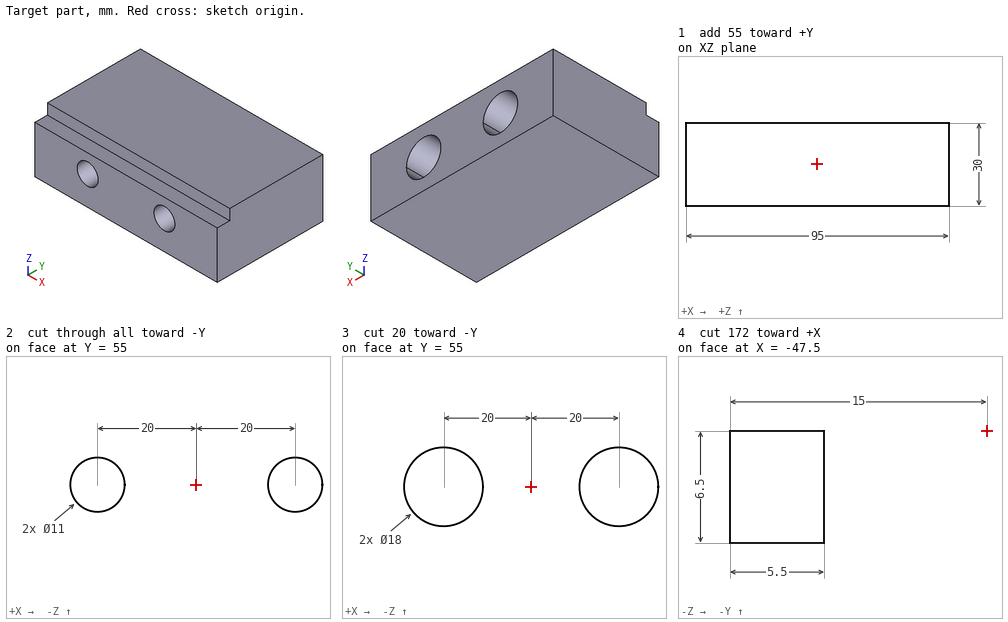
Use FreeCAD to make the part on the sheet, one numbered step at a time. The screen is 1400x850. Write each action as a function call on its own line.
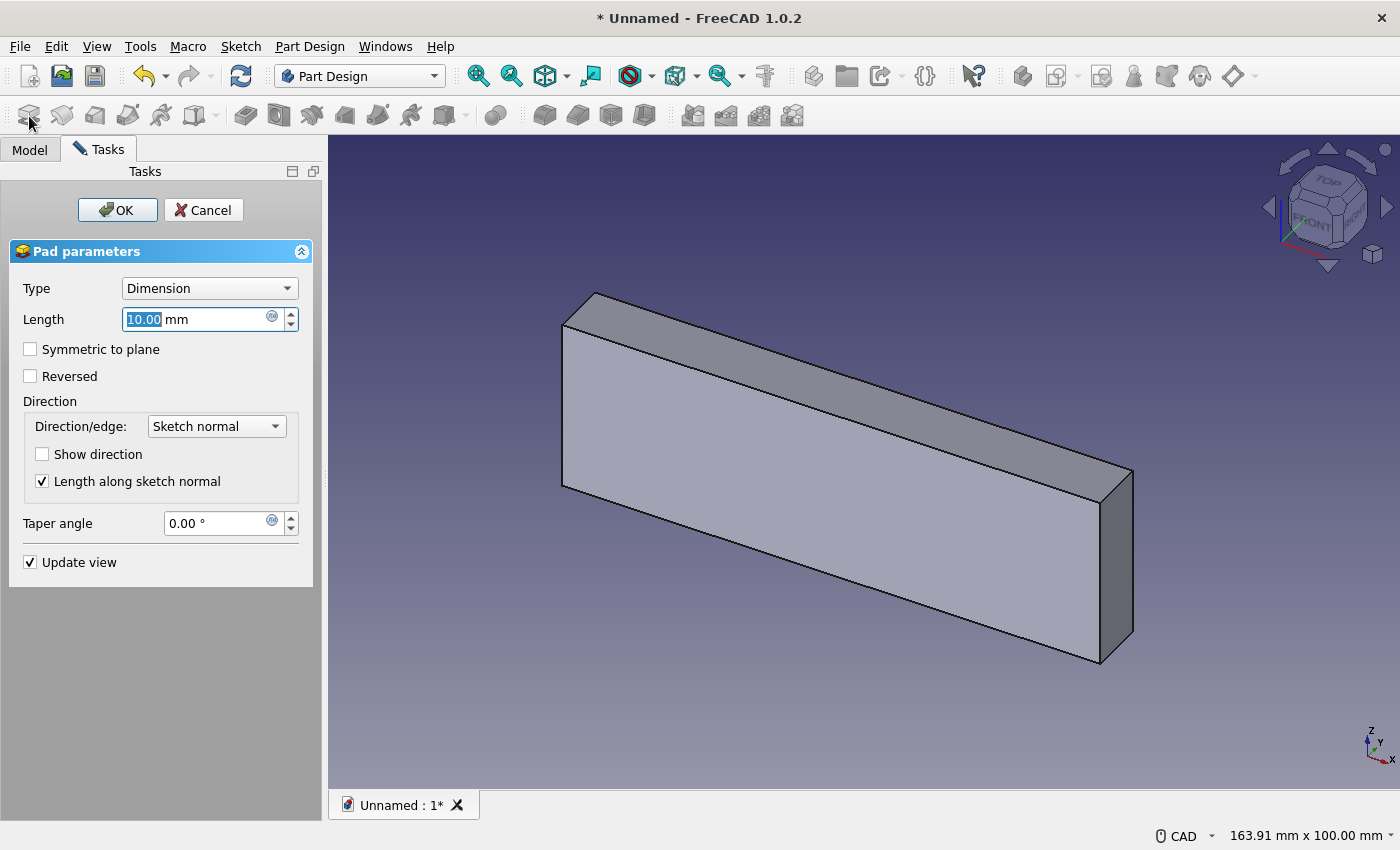
text(55)
key(Tab)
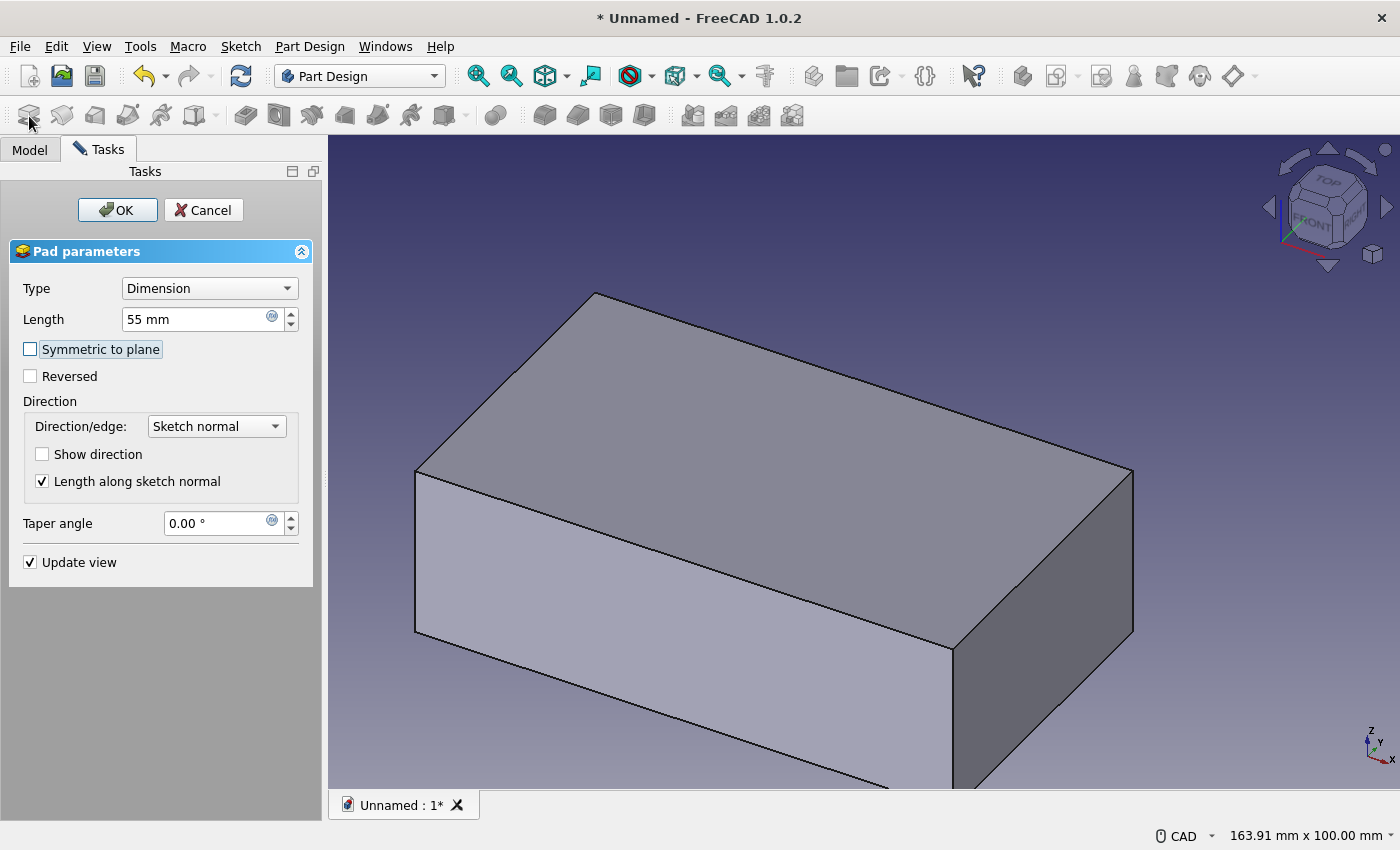
click(31, 376)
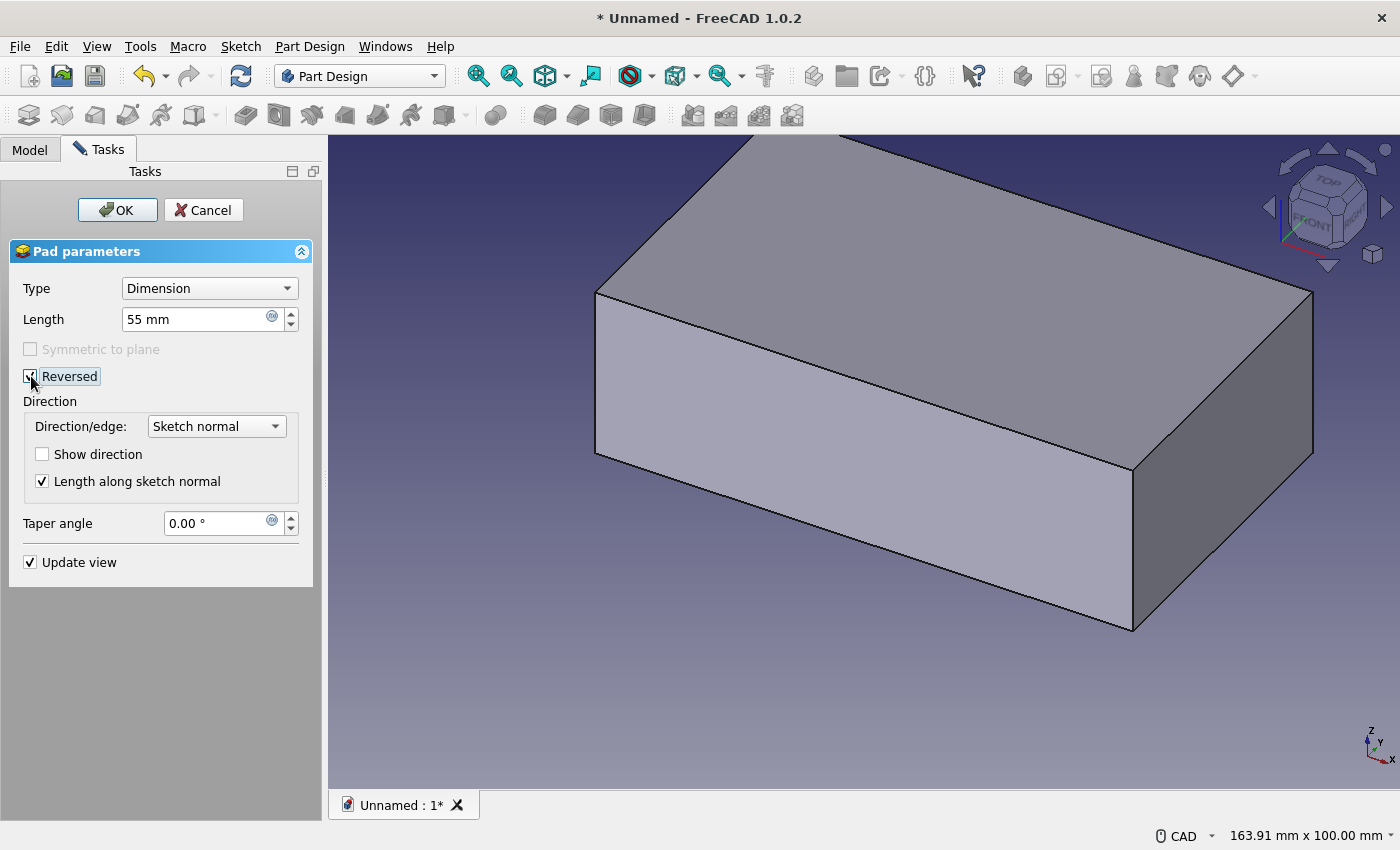
click(118, 210)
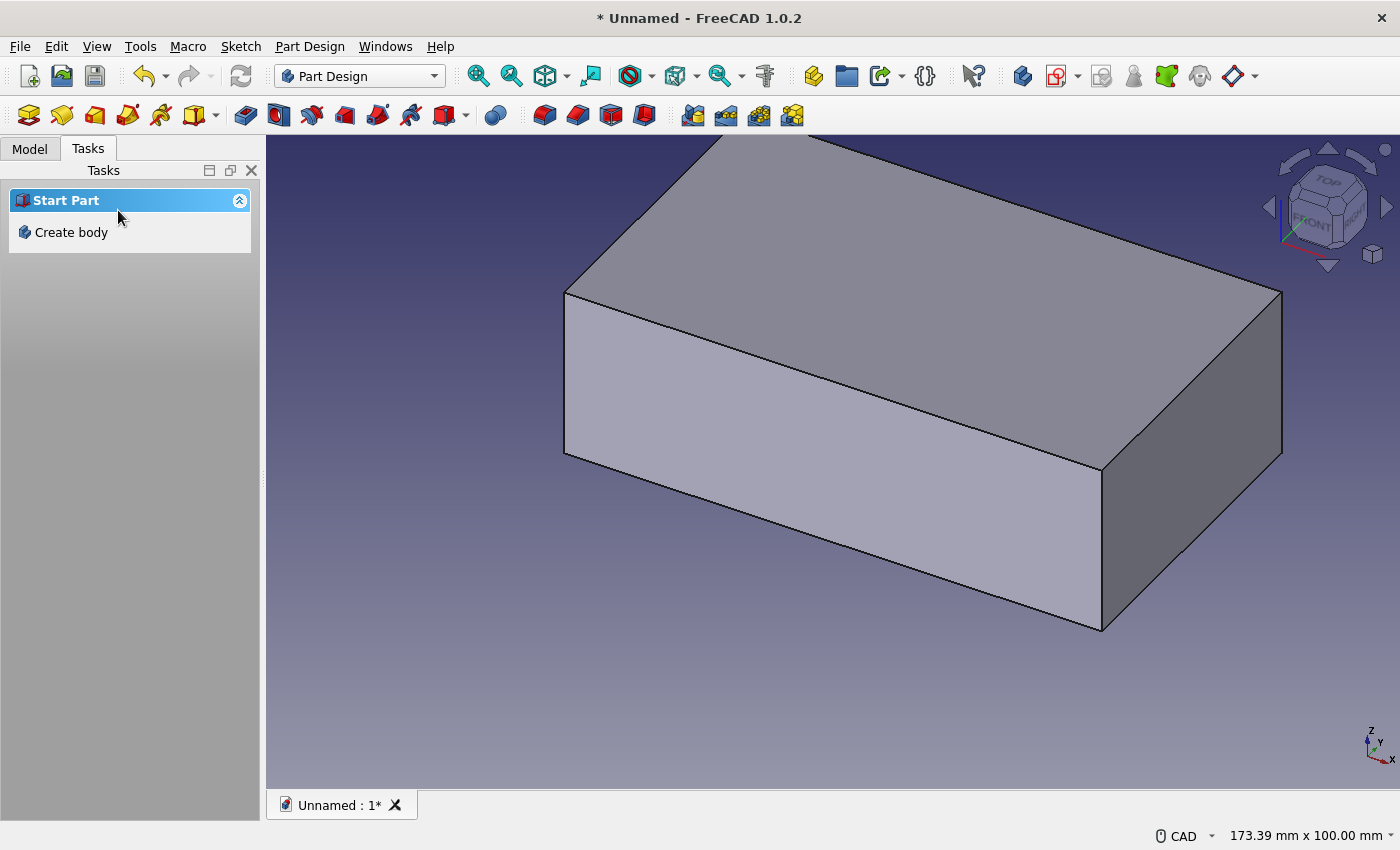
click(479, 76)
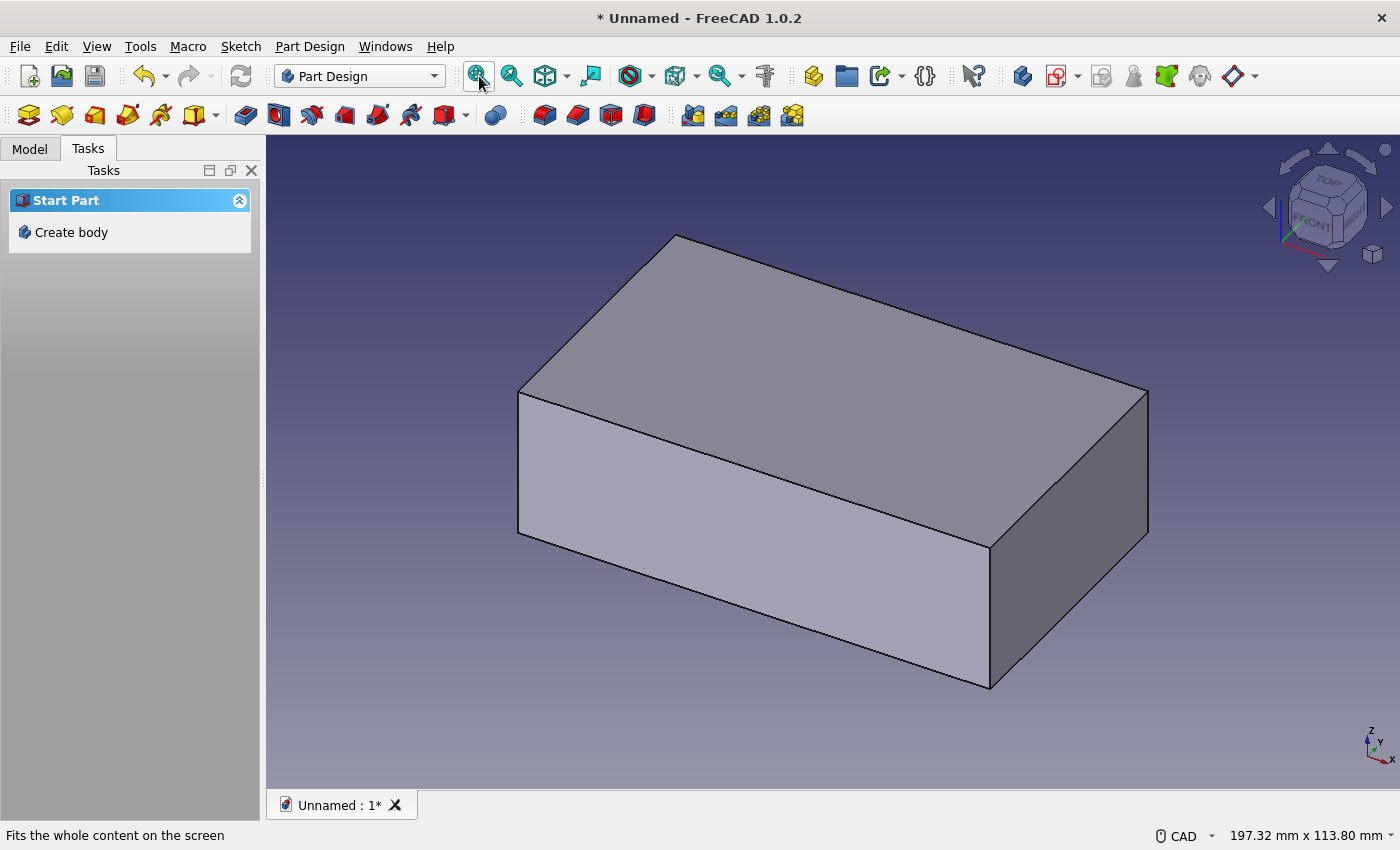
key(4)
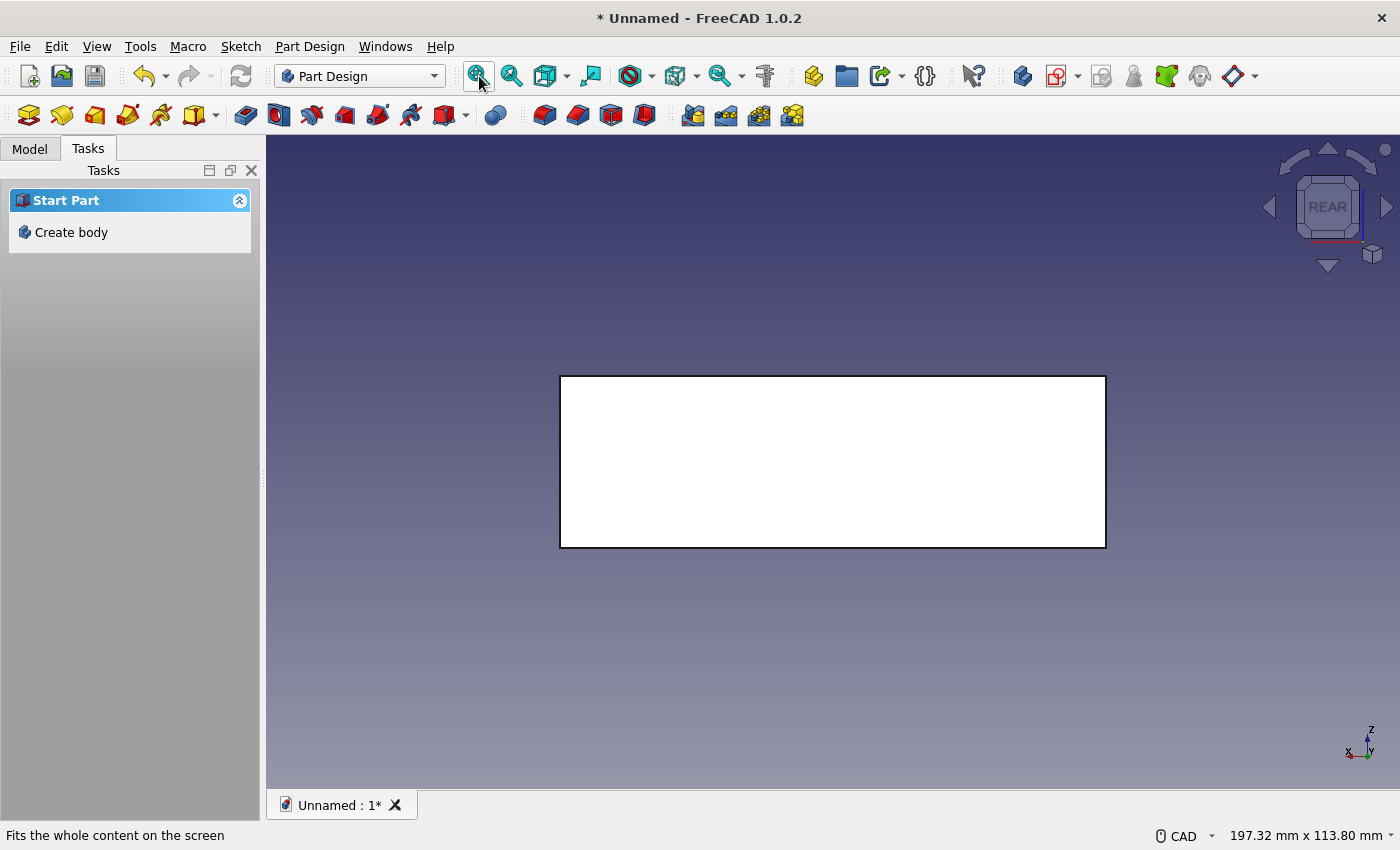
click(677, 461)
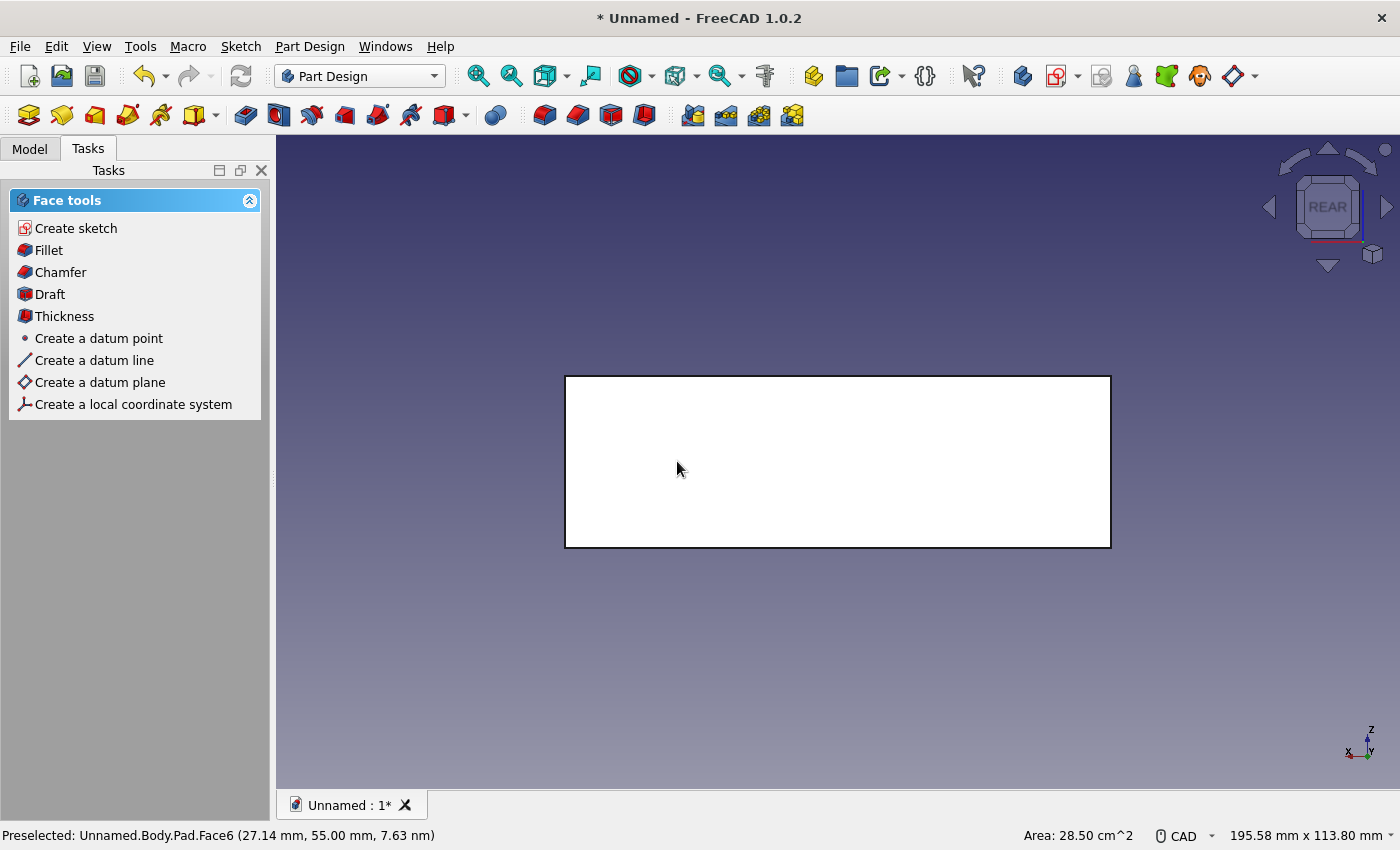
click(1056, 76)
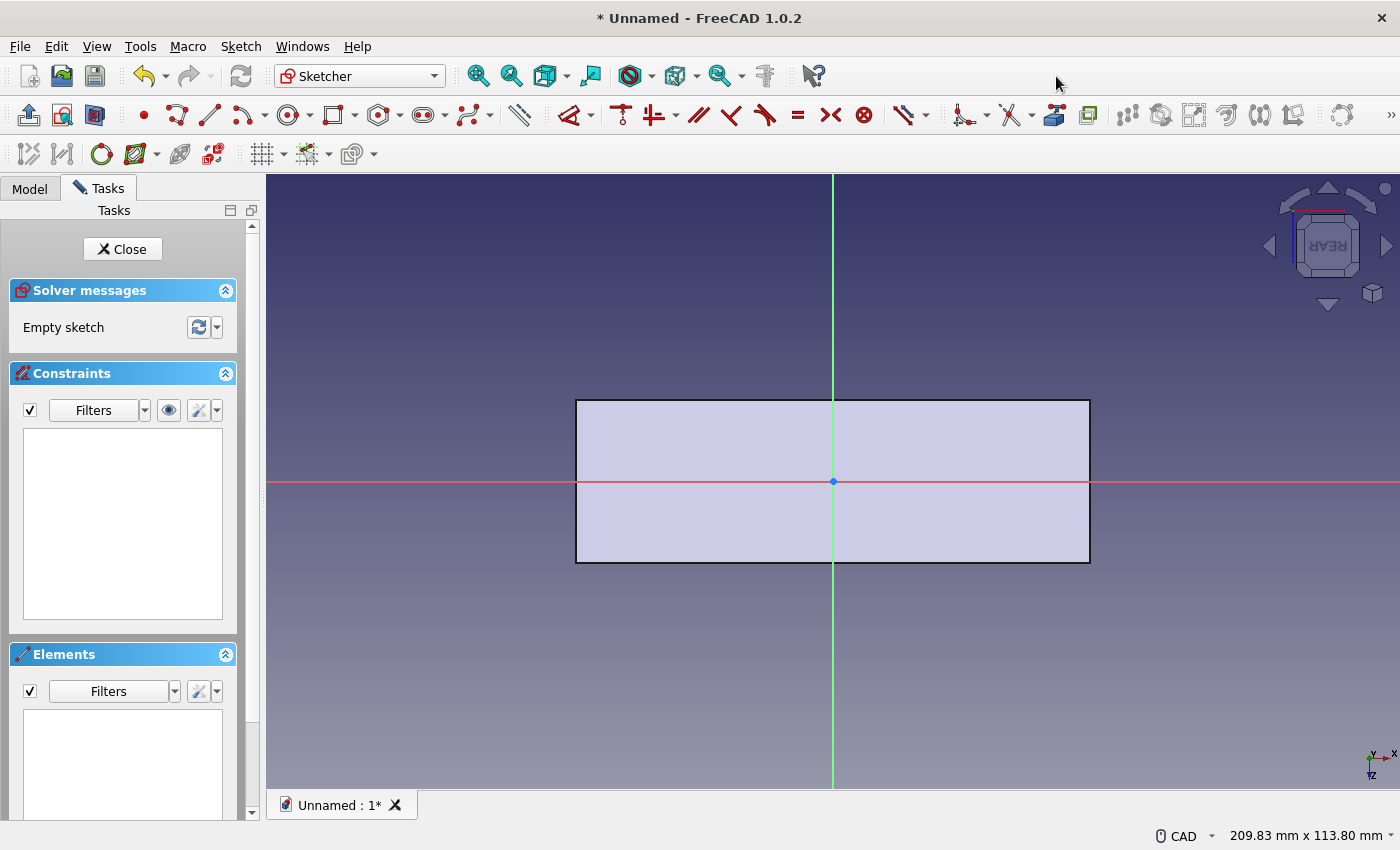
scroll(889, 481, up, 4)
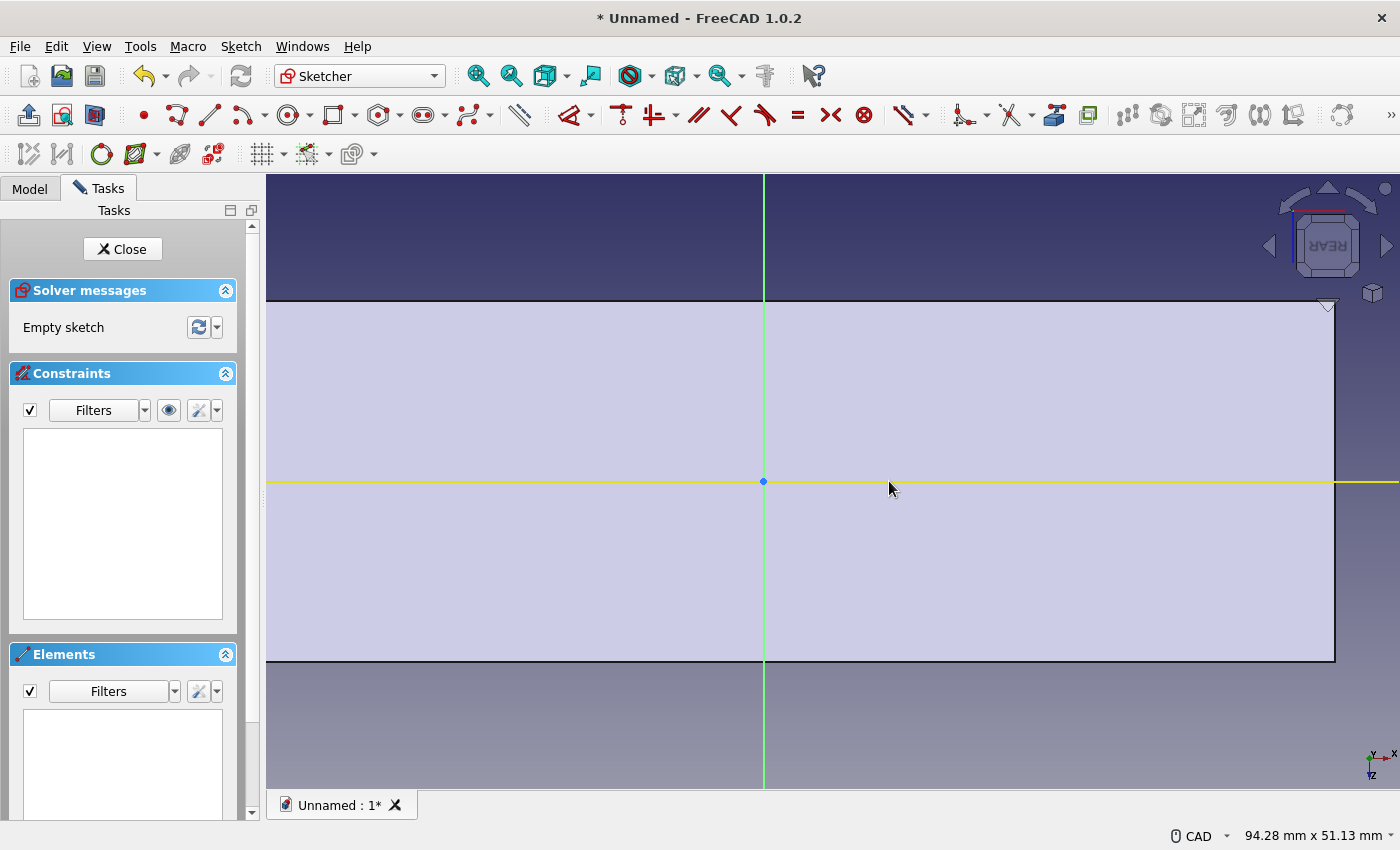
click(288, 116)